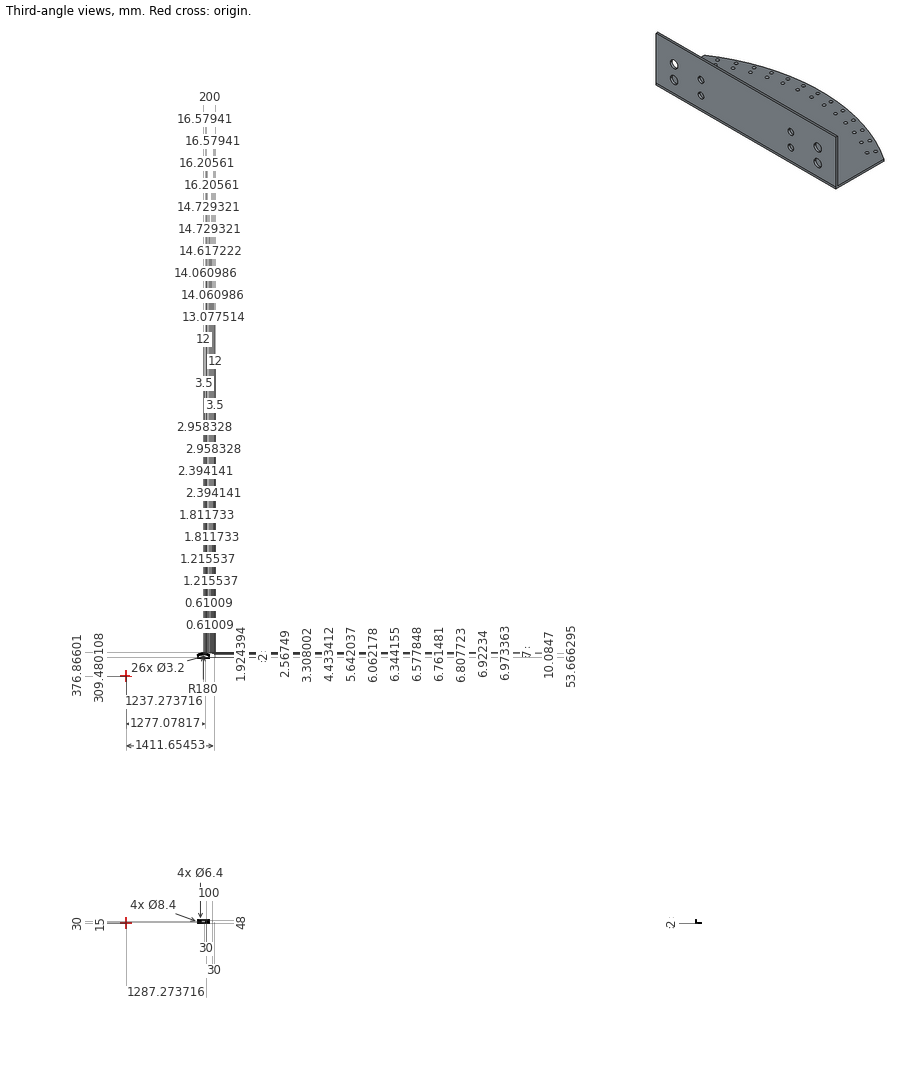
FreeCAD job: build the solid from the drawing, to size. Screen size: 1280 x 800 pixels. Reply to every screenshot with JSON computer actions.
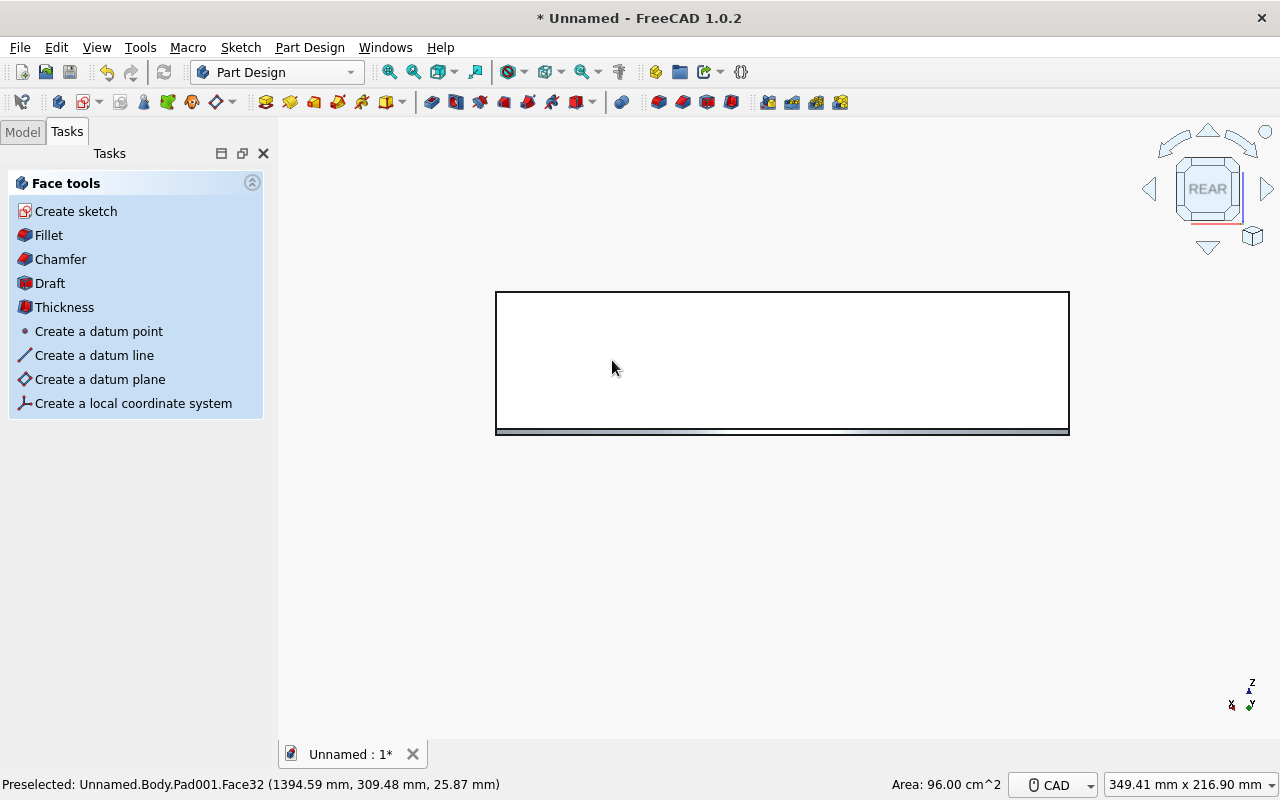
{"action": "left_click", "coordinate": [84, 102]}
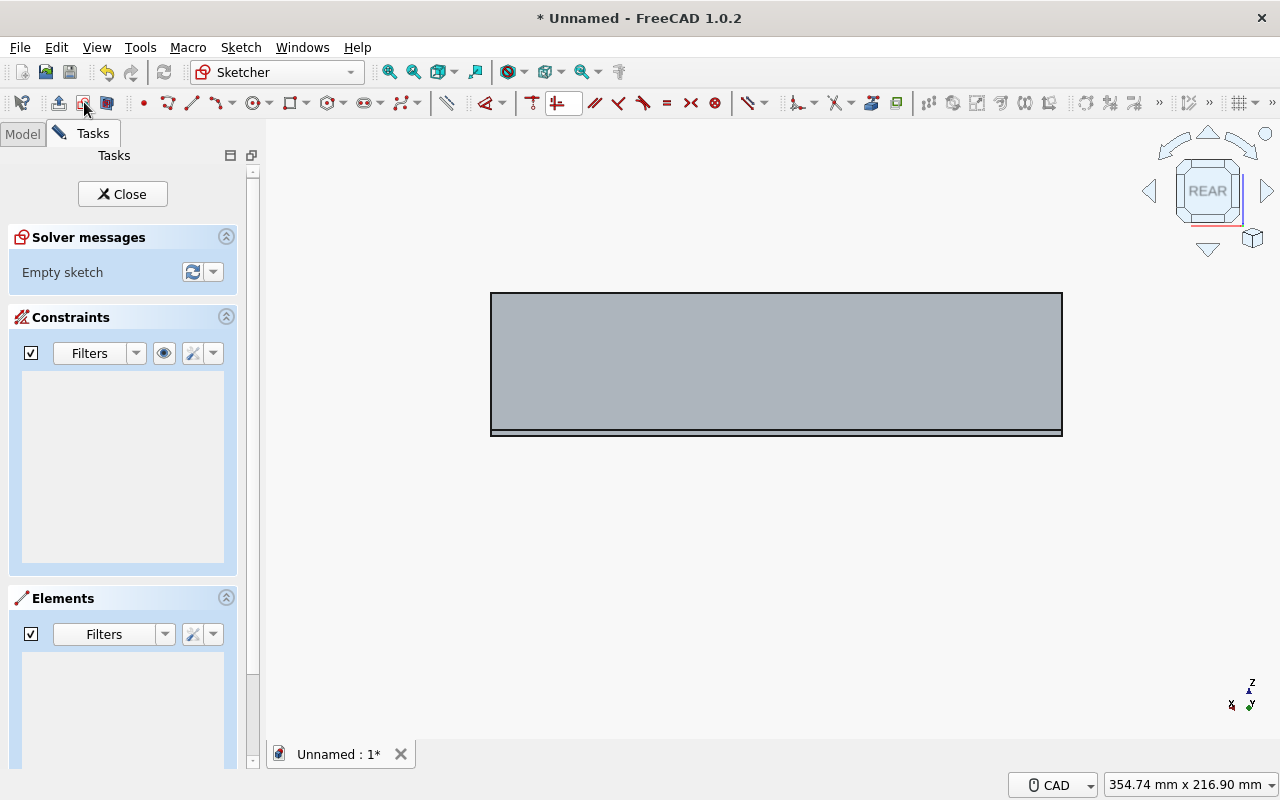
{"action": "key", "text": "q s"}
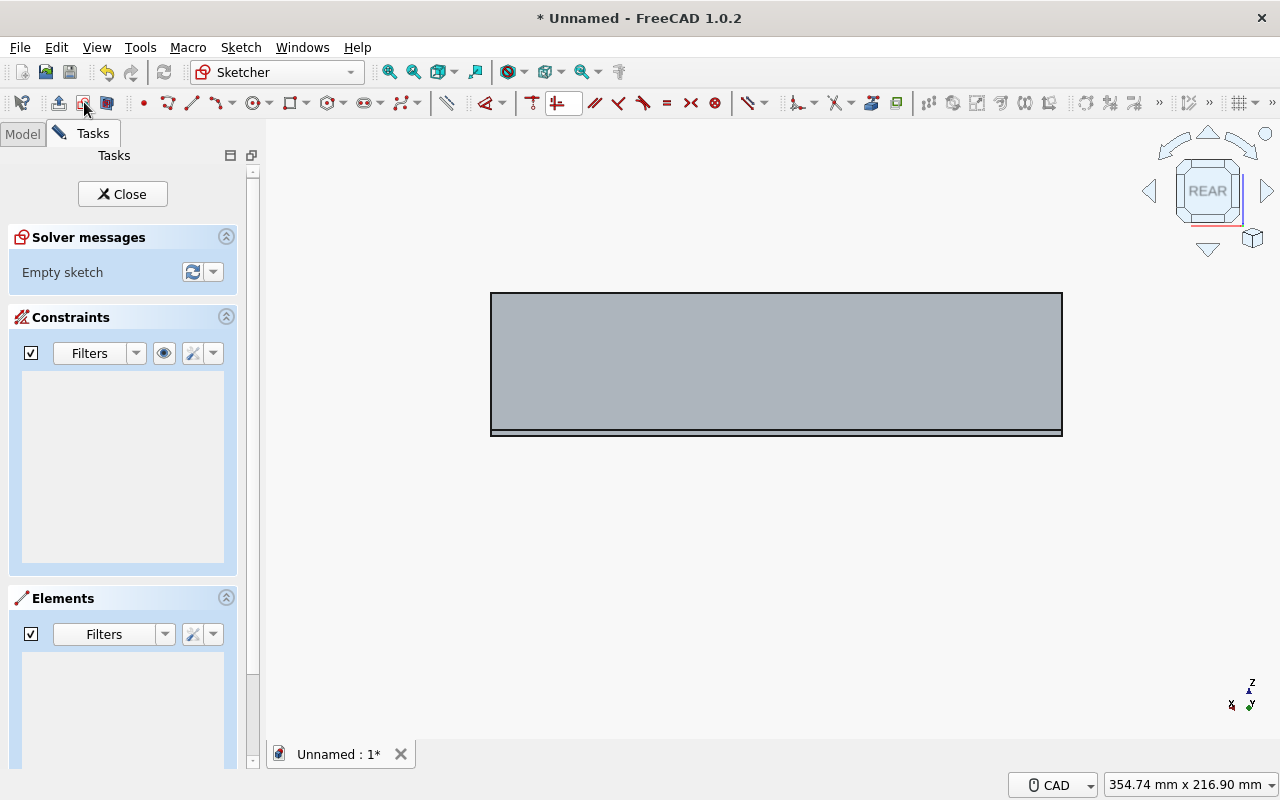
{"action": "key", "text": "g c"}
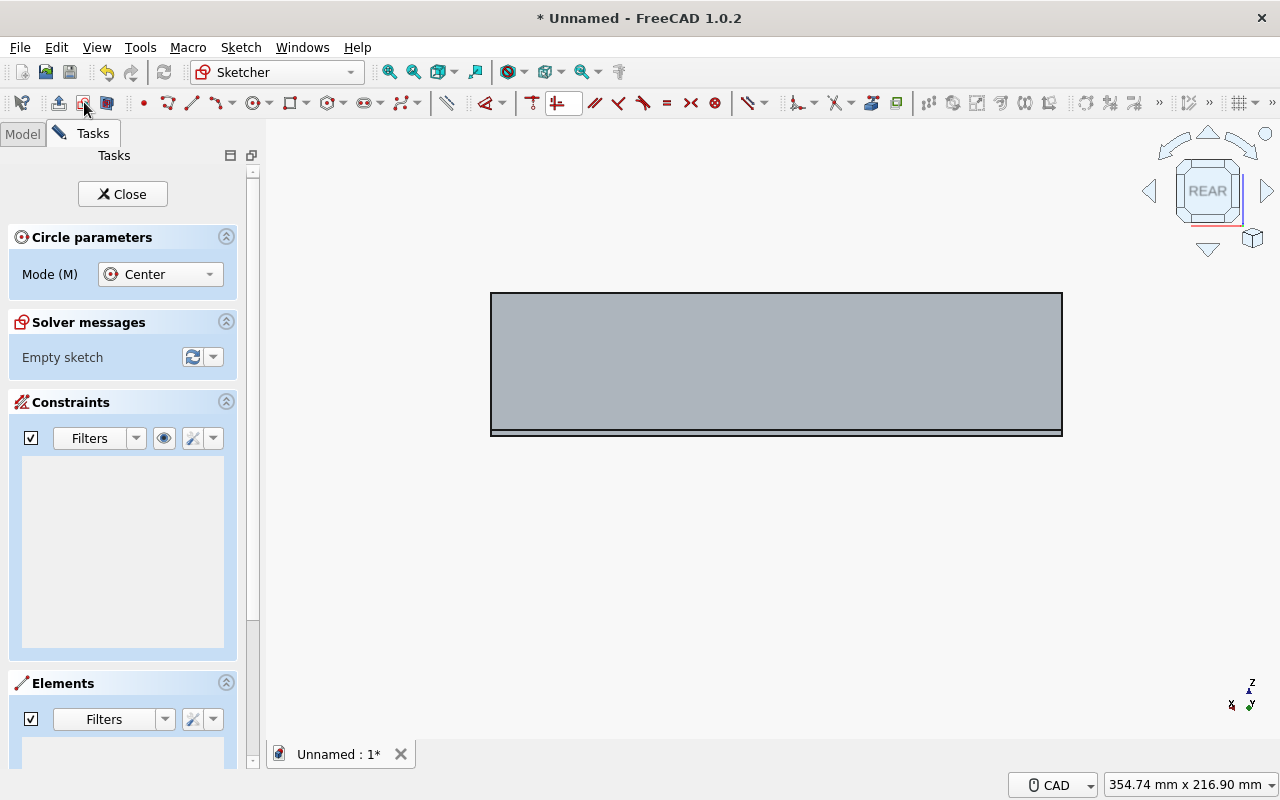
{"action": "scroll", "coordinate": [919, 350], "scroll_direction": "up", "scroll_amount": 5}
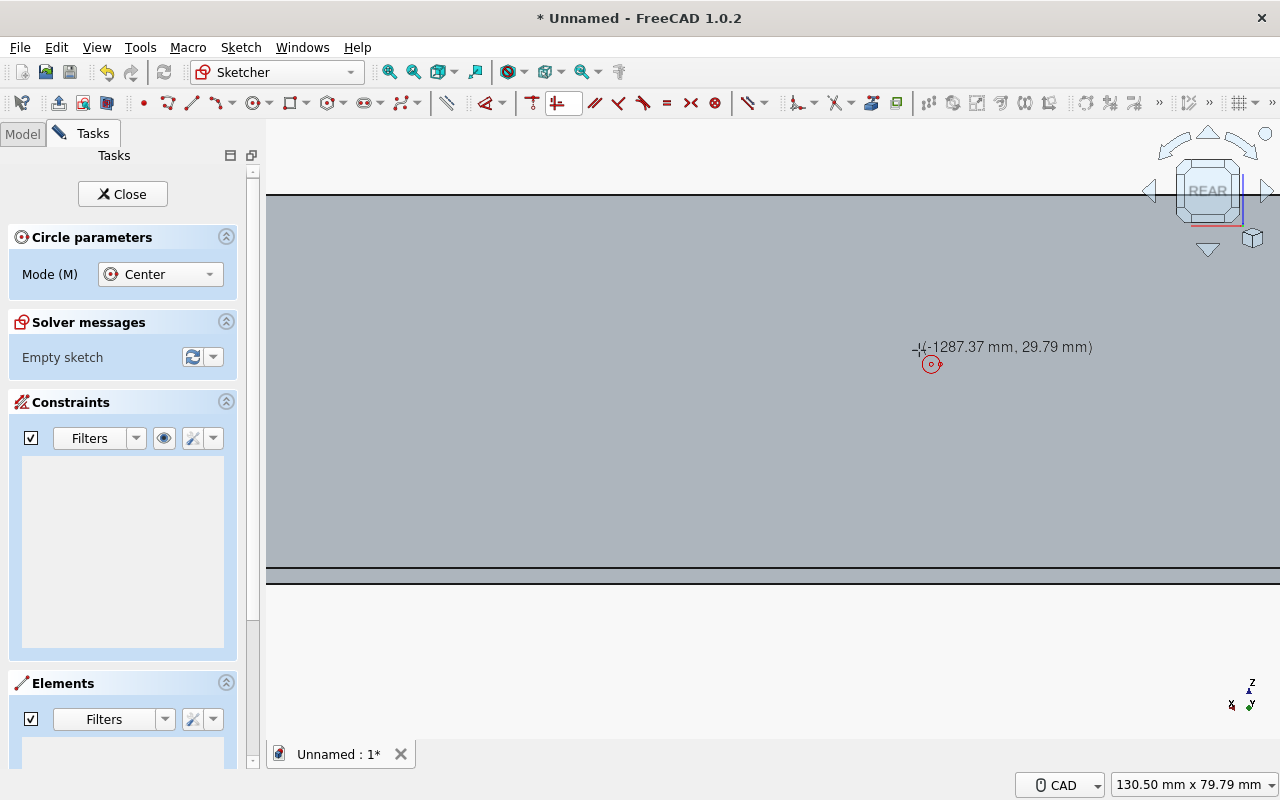
{"action": "left_click", "coordinate": [919, 350]}
{"action": "mouse_move", "coordinate": [936, 333]}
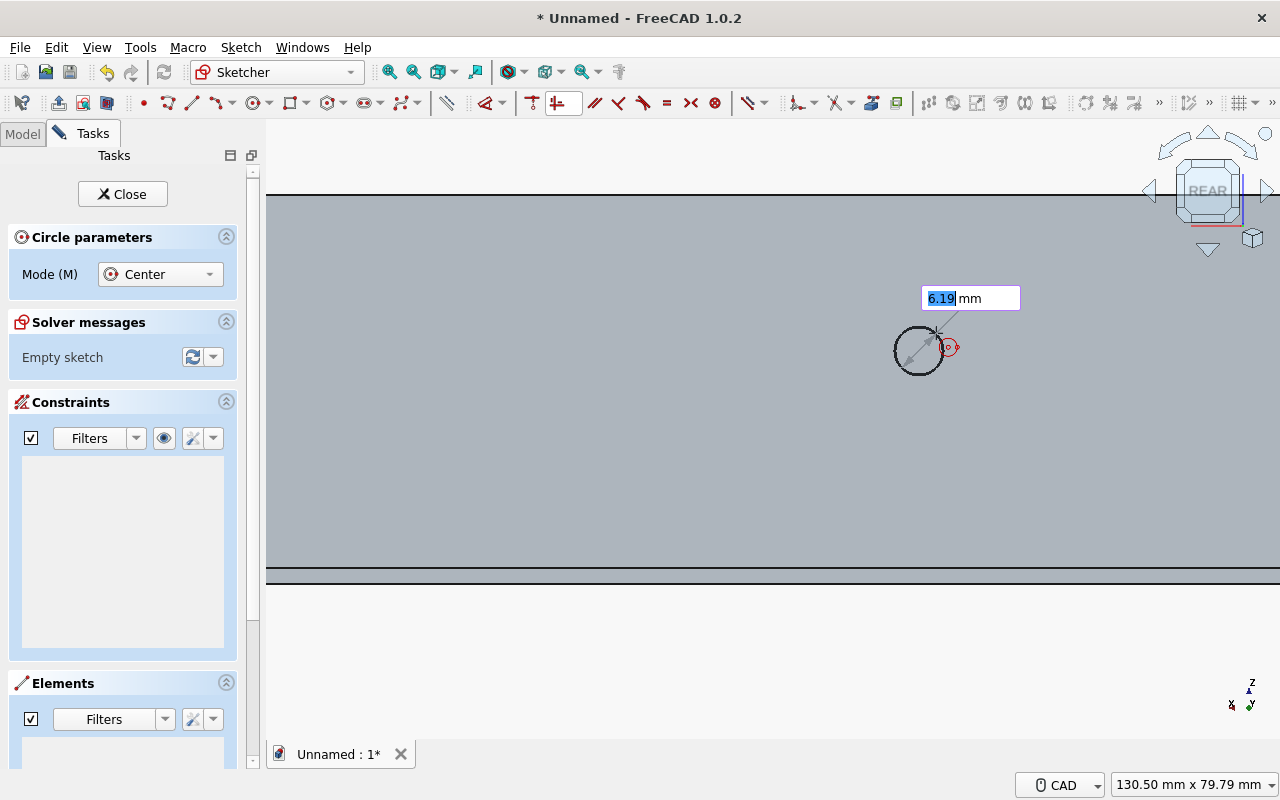
{"action": "type", "text": "6.4"}
{"action": "key", "text": "Return"}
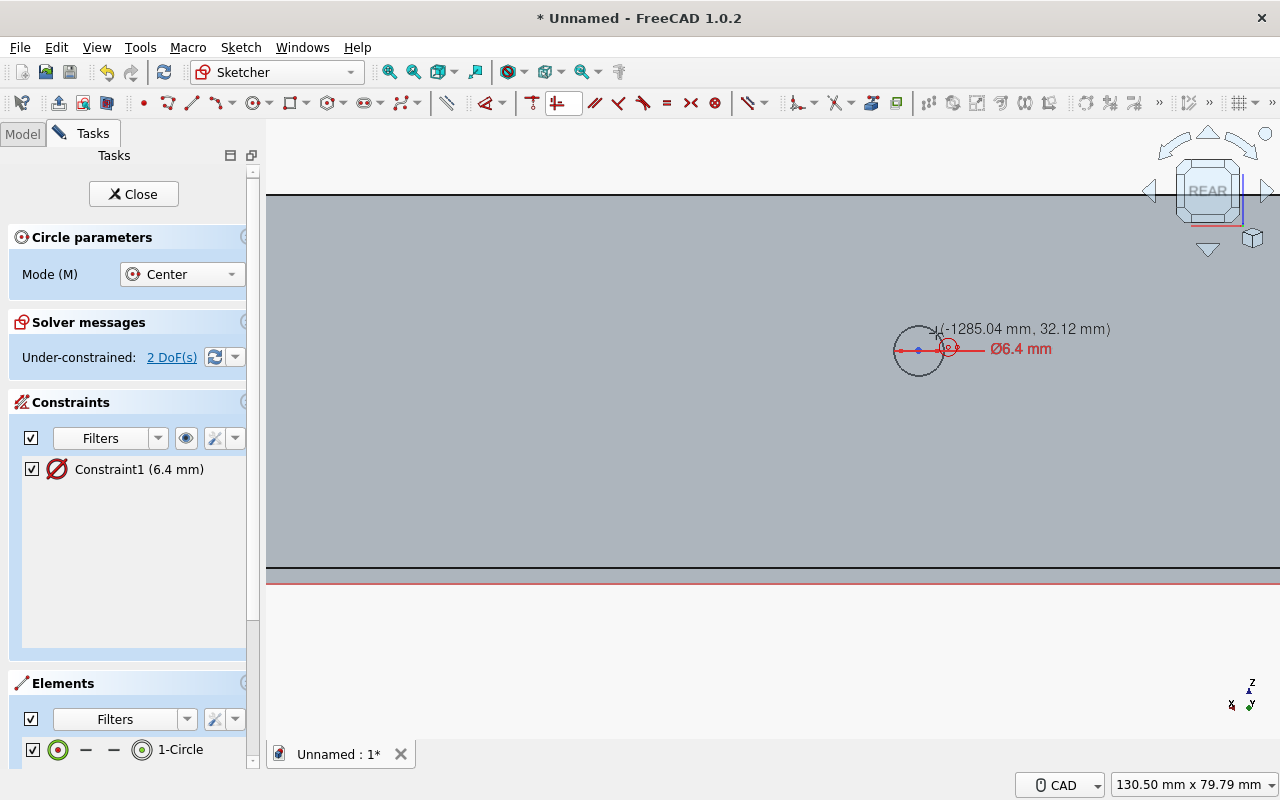
{"action": "scroll", "coordinate": [847, 446], "scroll_direction": "down", "scroll_amount": 4}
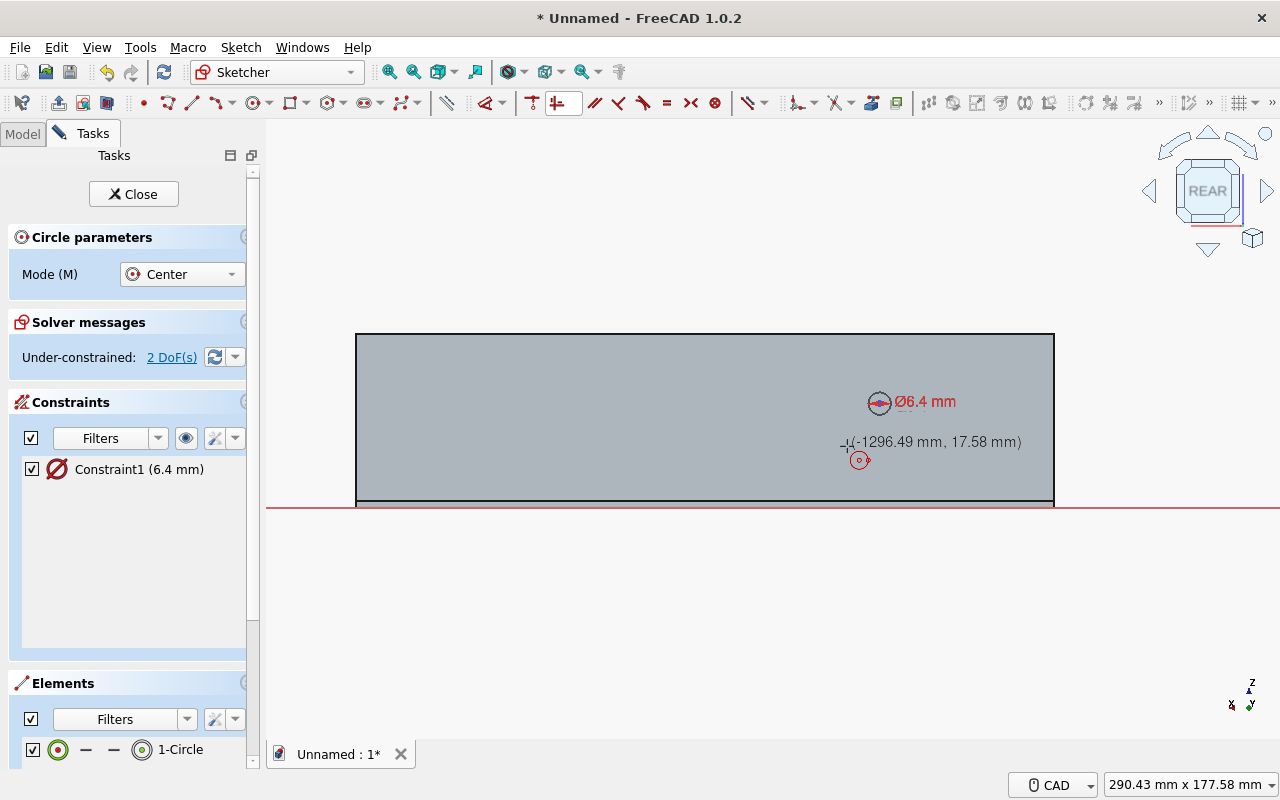
{"action": "scroll", "coordinate": [530, 403], "scroll_direction": "up", "scroll_amount": 4}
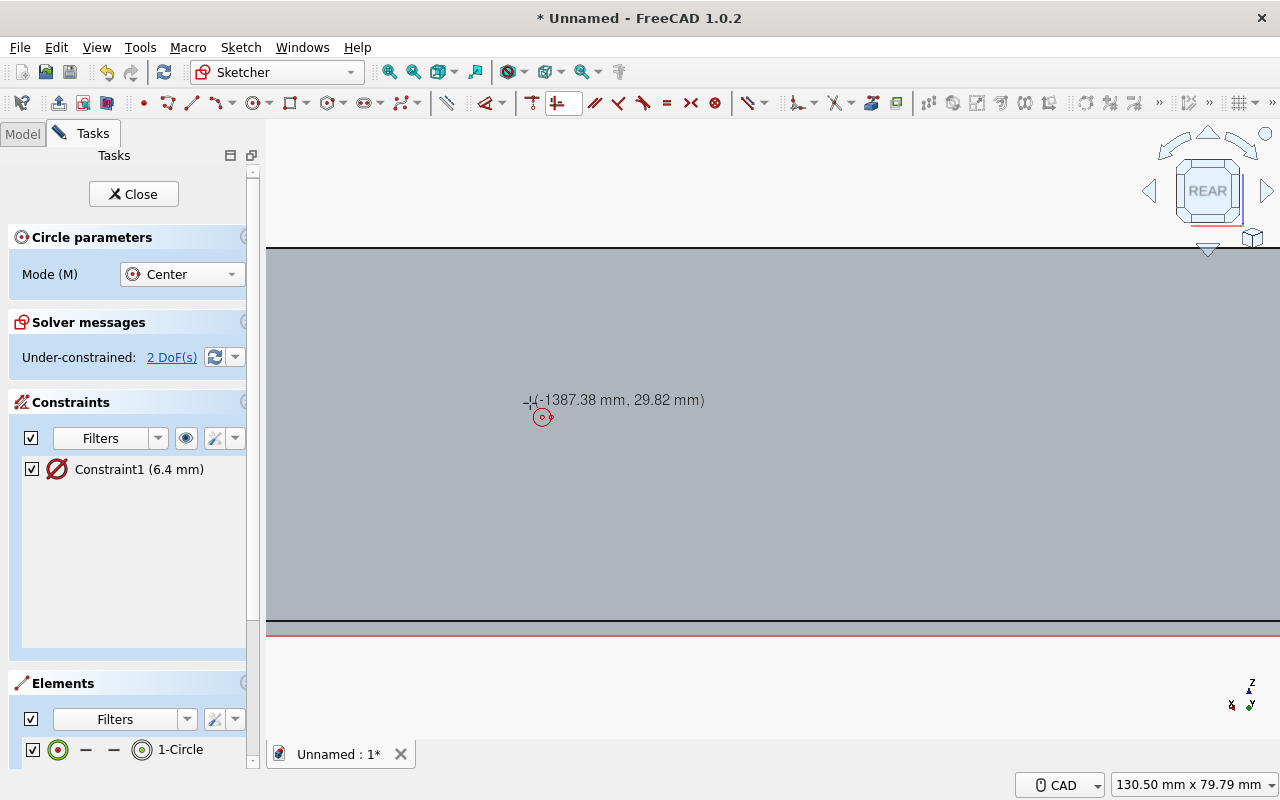
{"action": "left_click", "coordinate": [531, 403]}
{"action": "mouse_move", "coordinate": [548, 386]}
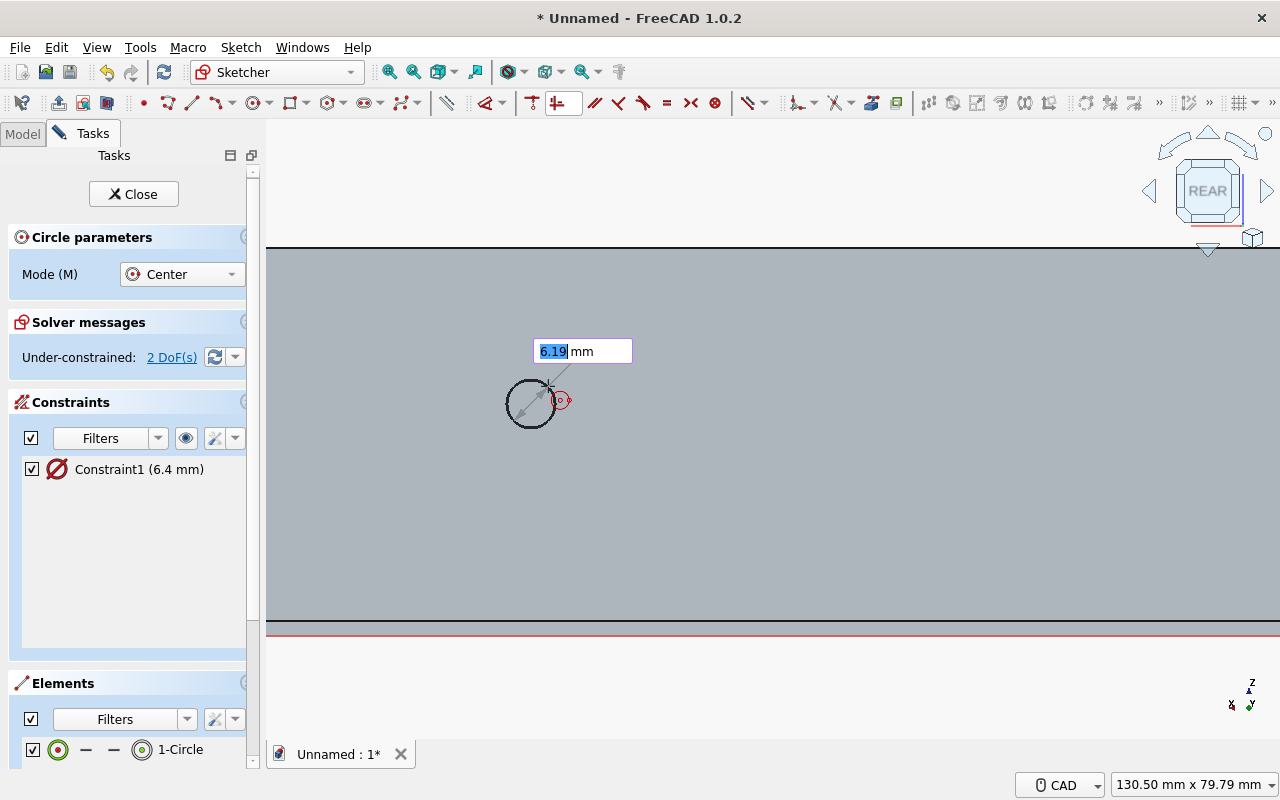
{"action": "type", "text": "6.4"}
{"action": "key", "text": "Return"}